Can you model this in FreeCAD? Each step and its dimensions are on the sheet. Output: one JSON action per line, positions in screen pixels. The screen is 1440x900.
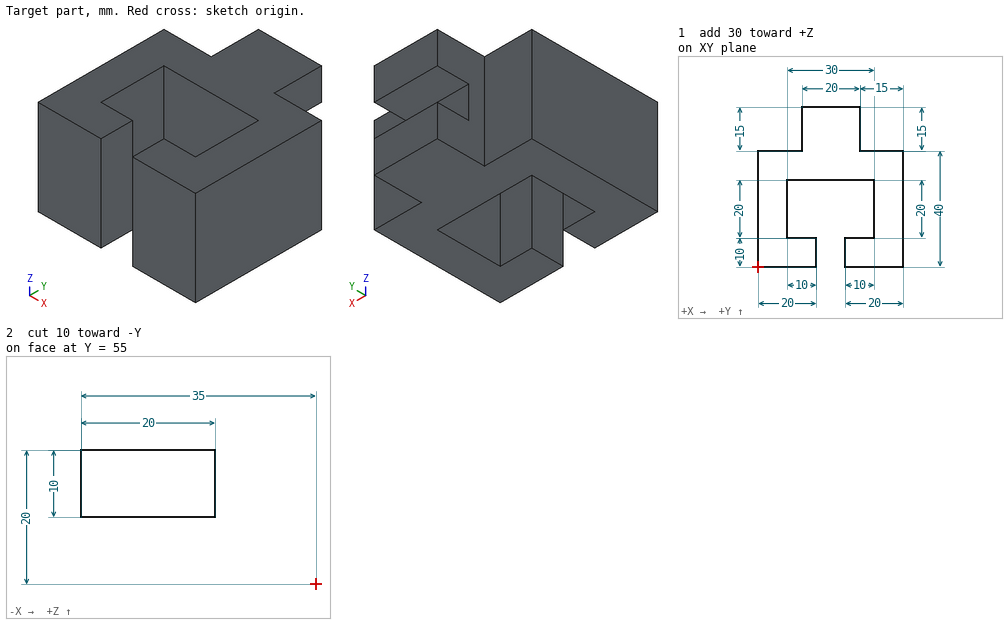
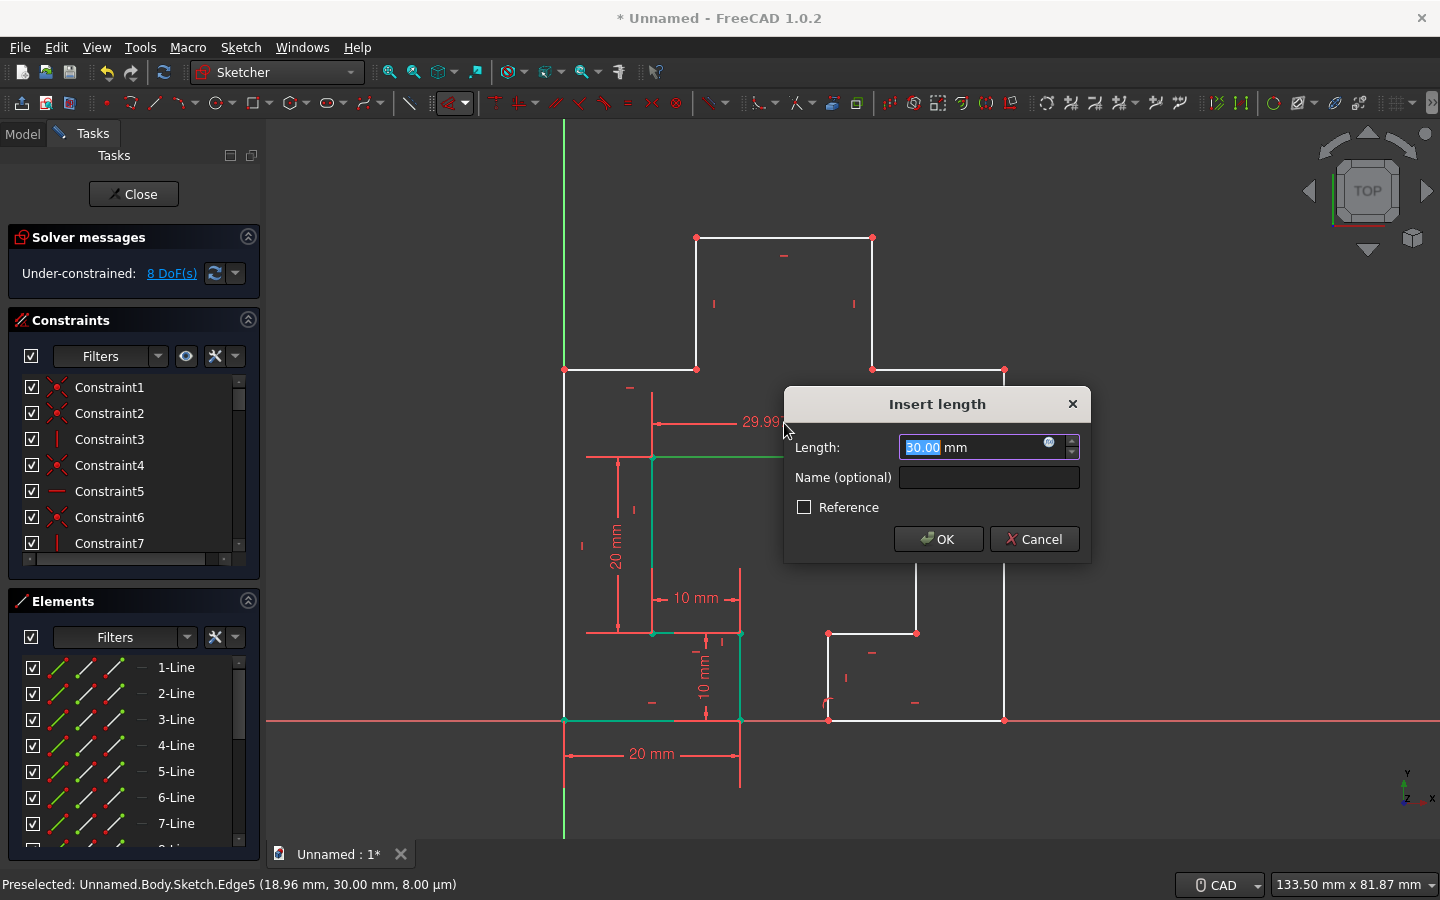
{"action": "type", "text": "30"}
{"action": "key", "text": "Return"}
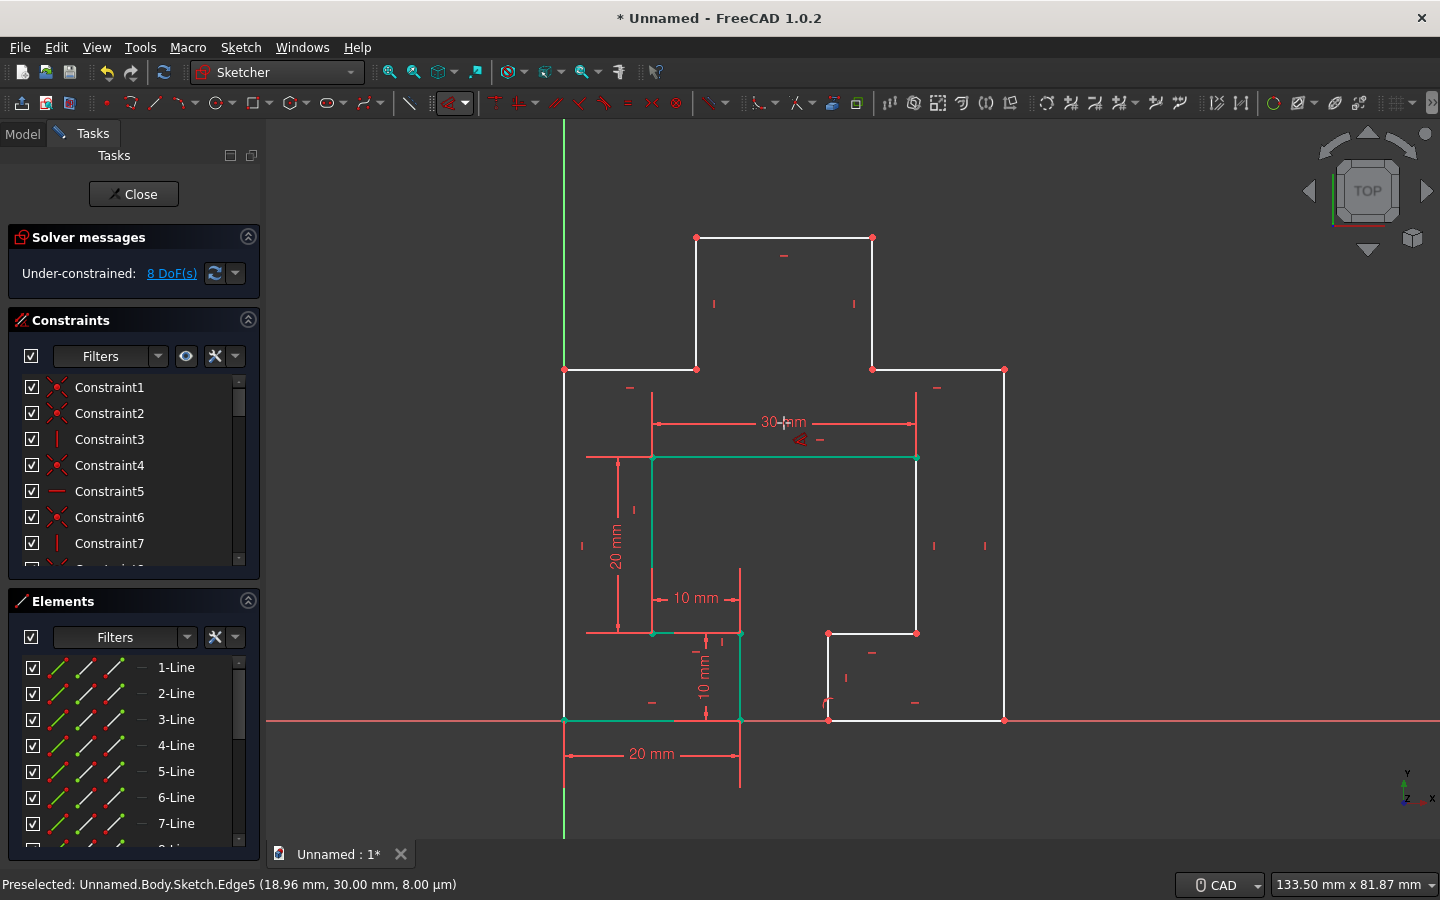
{"action": "left_click", "coordinate": [916, 510]}
{"action": "left_click", "coordinate": [950, 546]}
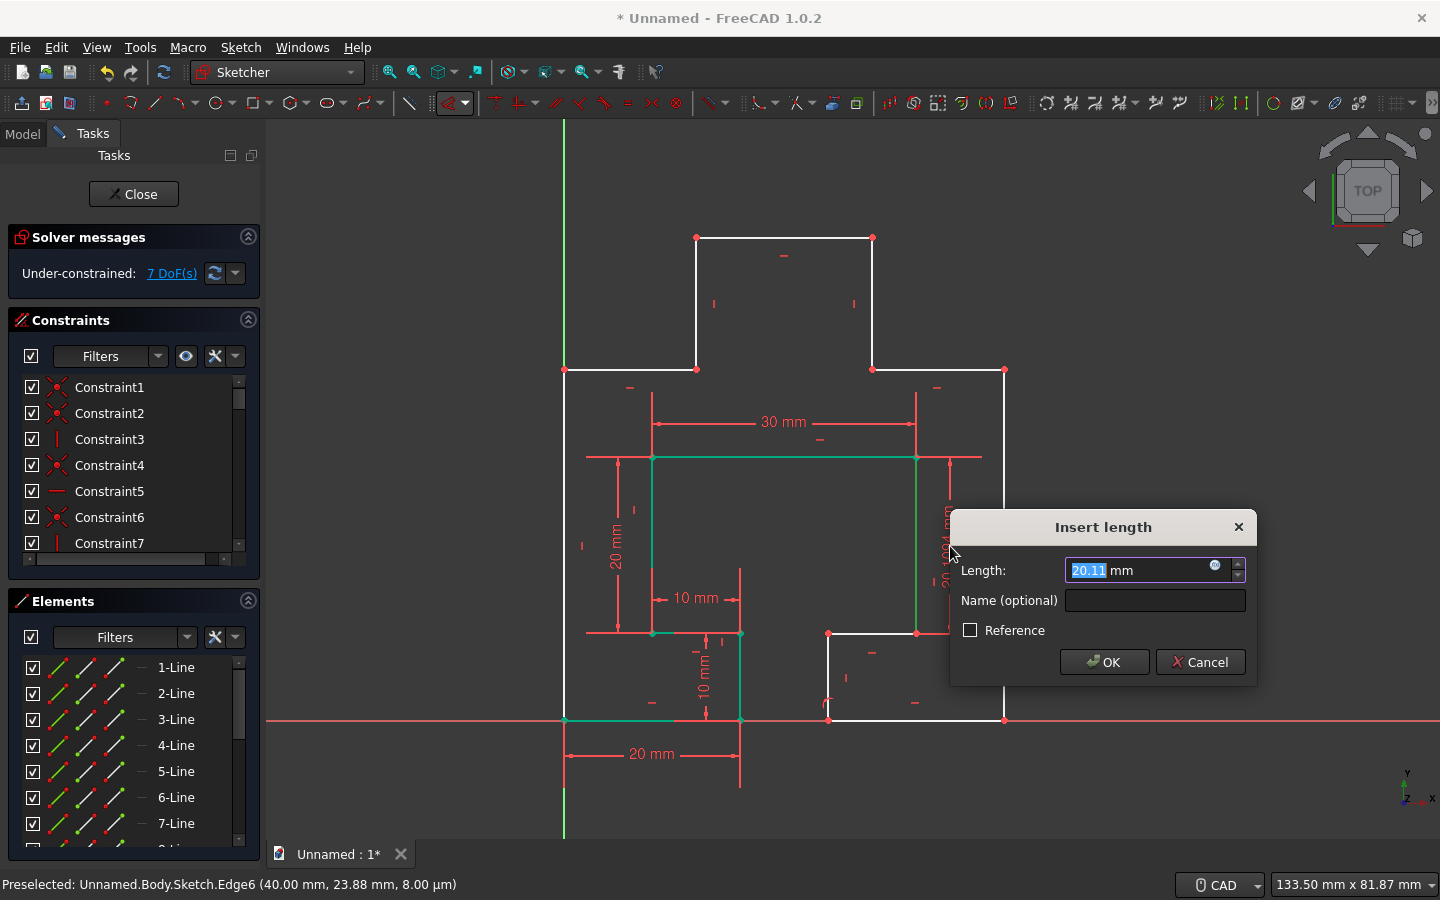
{"action": "type", "text": "20"}
{"action": "key", "text": "Return"}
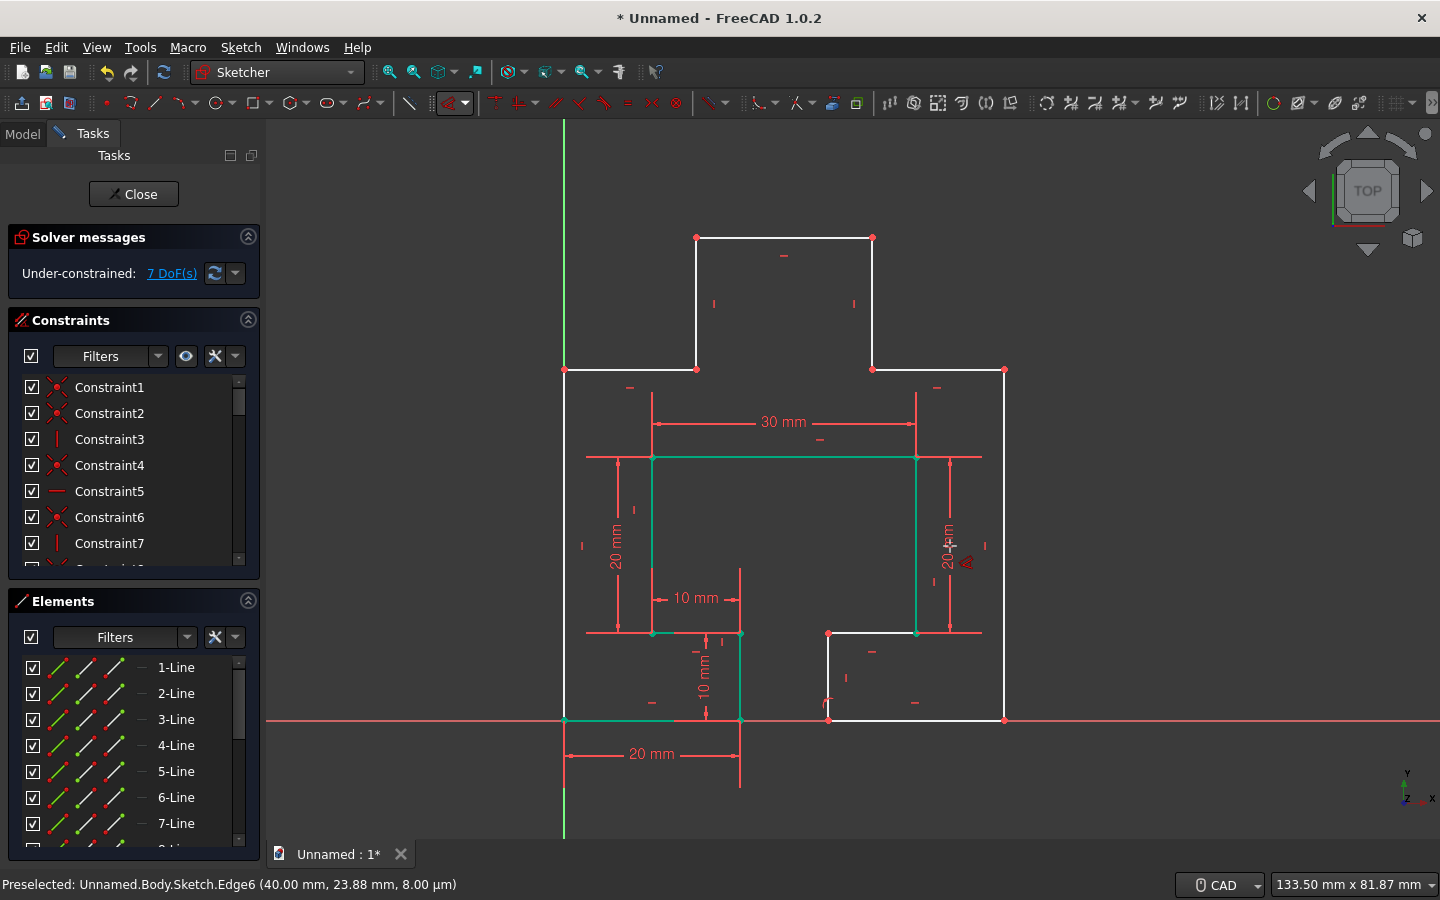
{"action": "left_click", "coordinate": [890, 633]}
{"action": "left_click", "coordinate": [872, 667]}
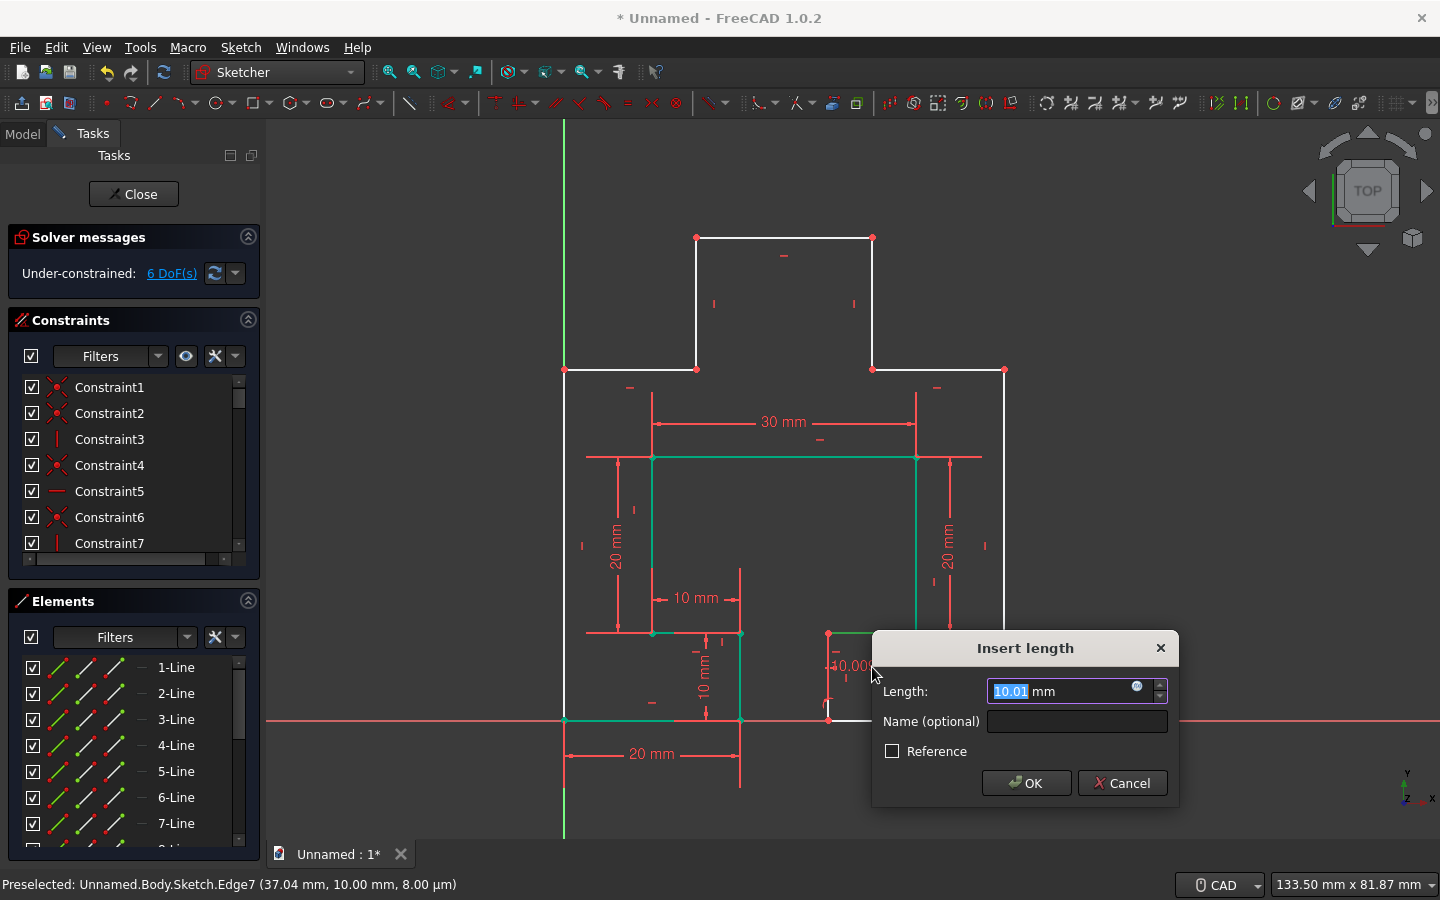
{"action": "type", "text": "10"}
{"action": "key", "text": "Return"}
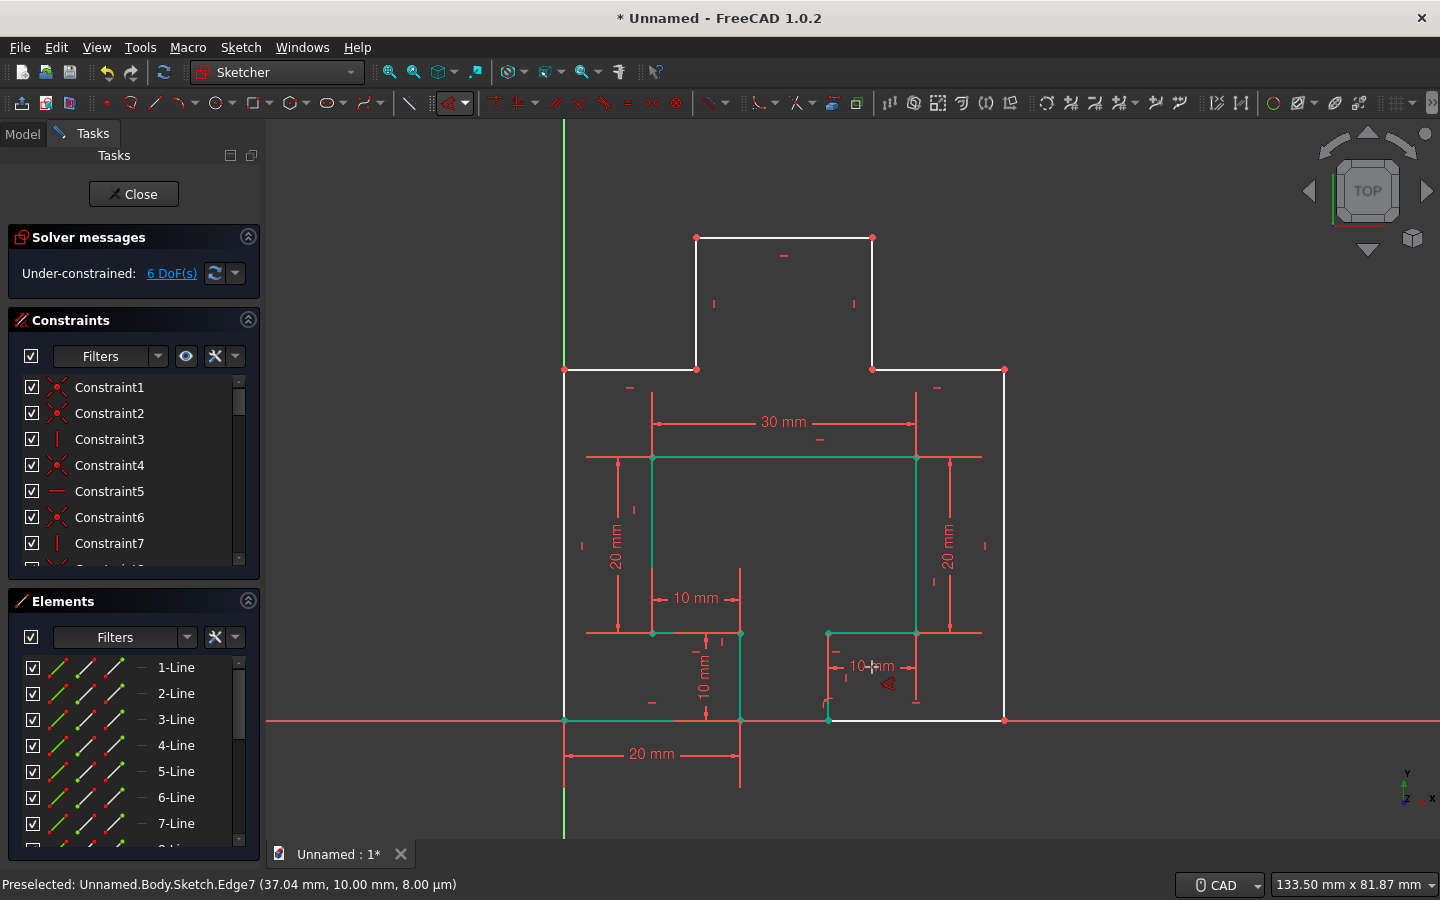
{"action": "left_click", "coordinate": [881, 721]}
{"action": "left_click", "coordinate": [916, 755]}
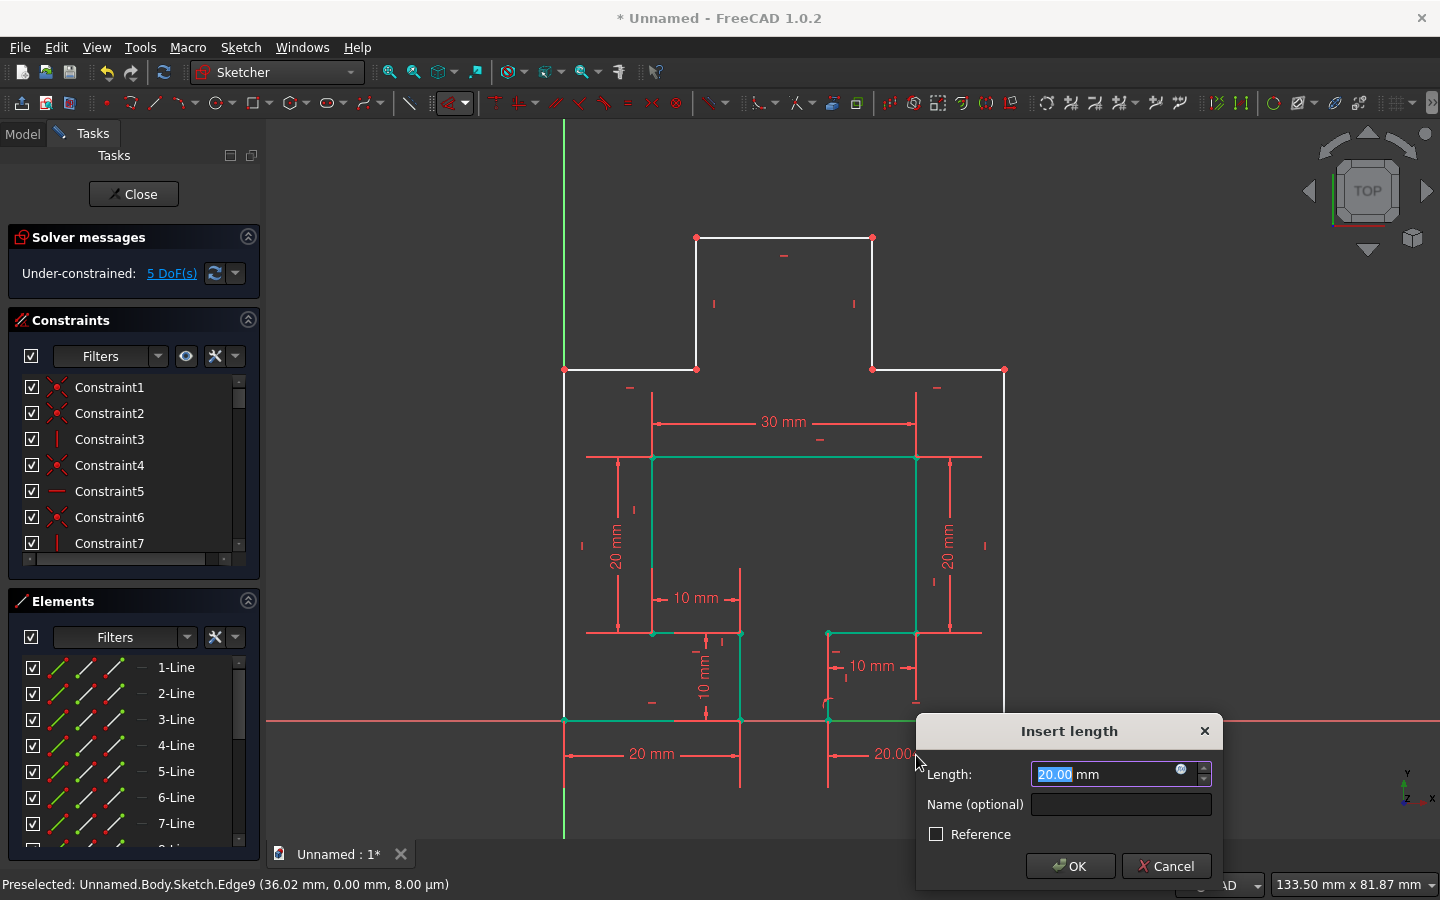
{"action": "type", "text": "20"}
{"action": "key", "text": "Return"}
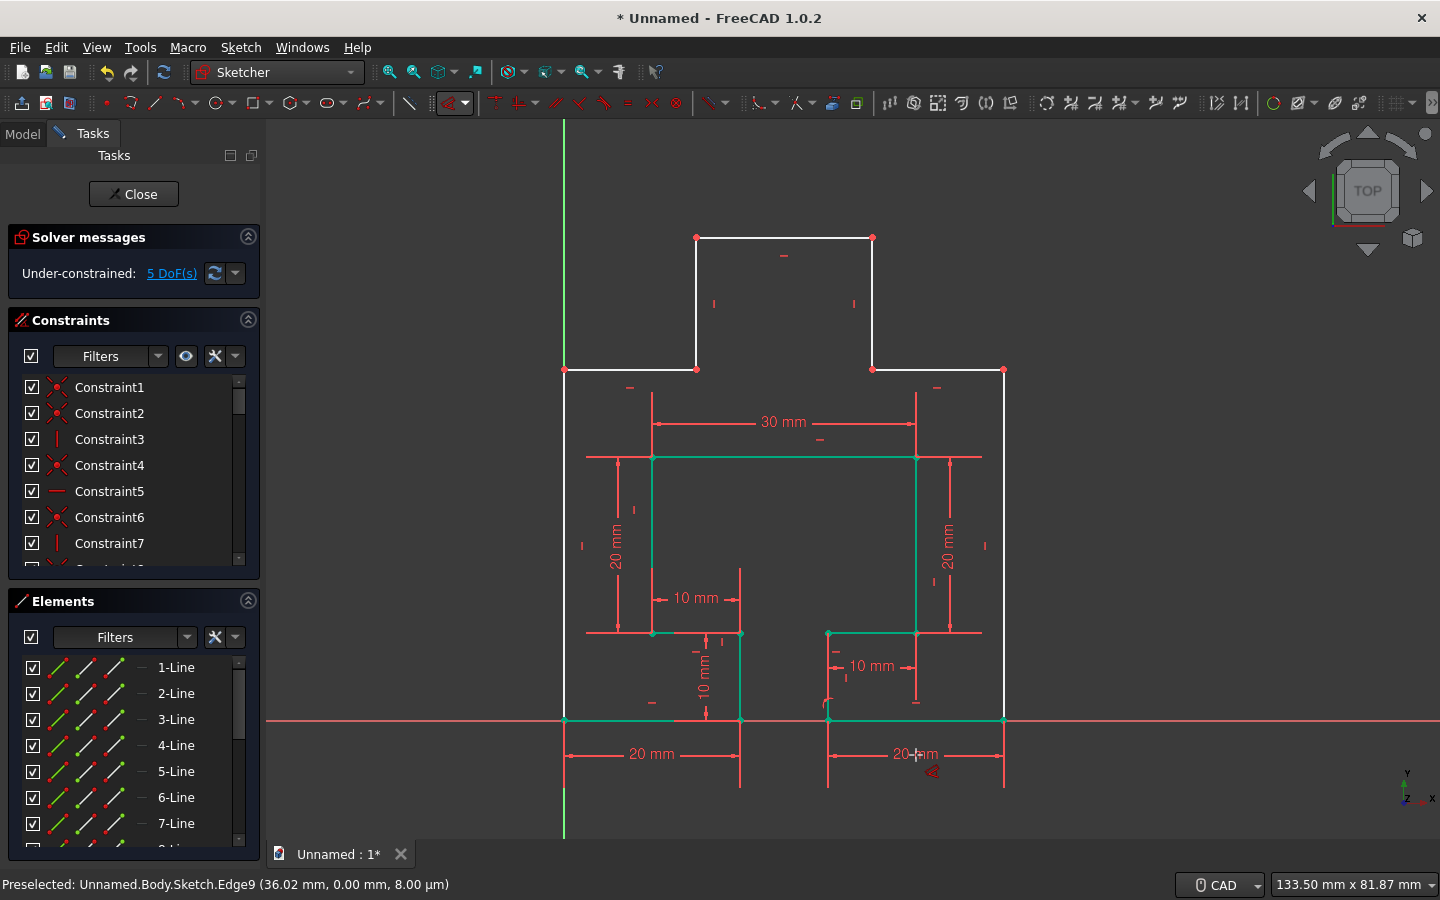
{"action": "left_click", "coordinate": [1004, 616]}
{"action": "left_click", "coordinate": [1038, 545]}